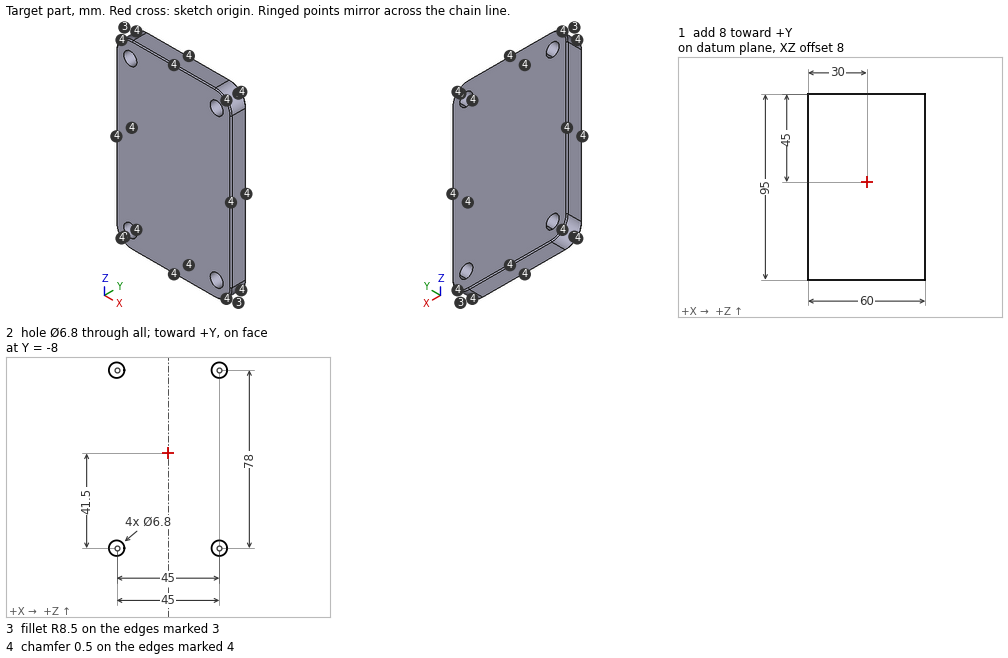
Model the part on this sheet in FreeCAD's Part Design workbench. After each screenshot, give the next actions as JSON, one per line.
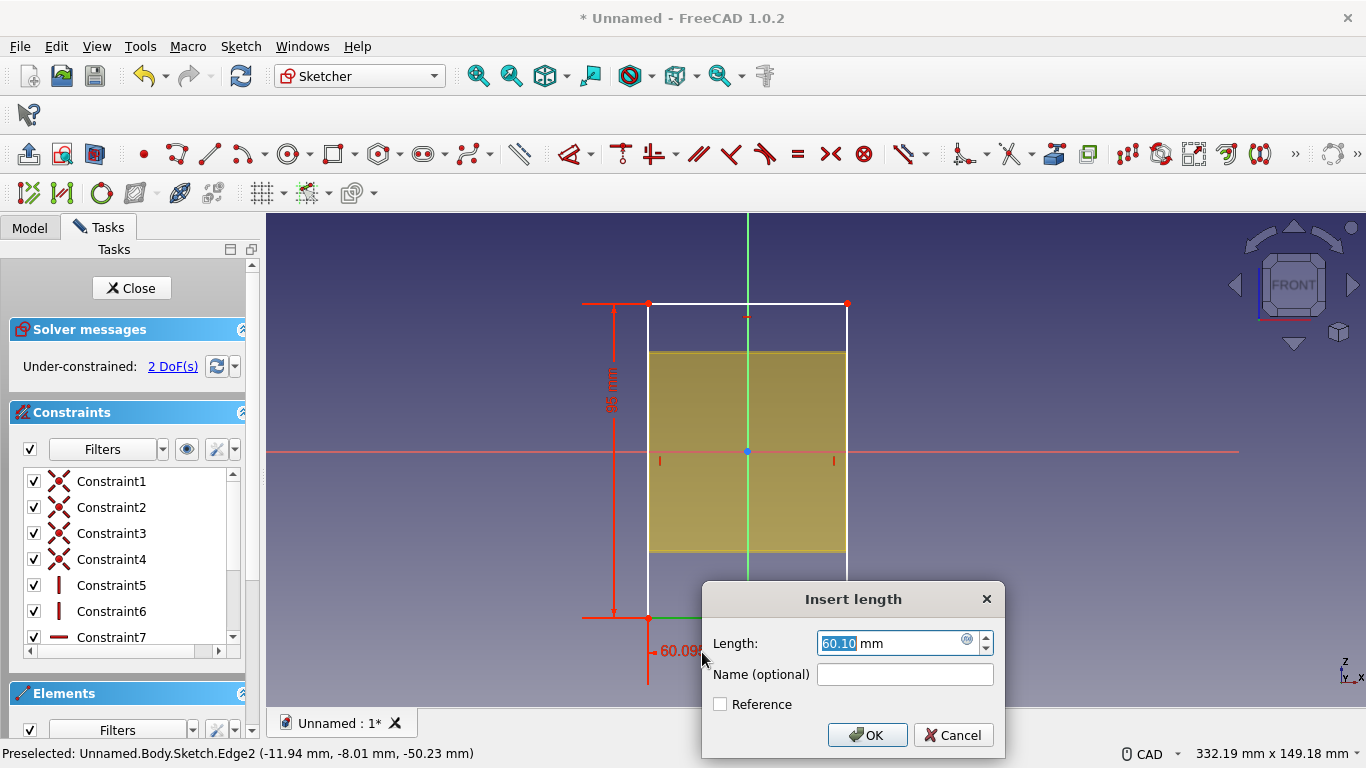
{"action": "type", "text": "60"}
{"action": "key", "text": "Return"}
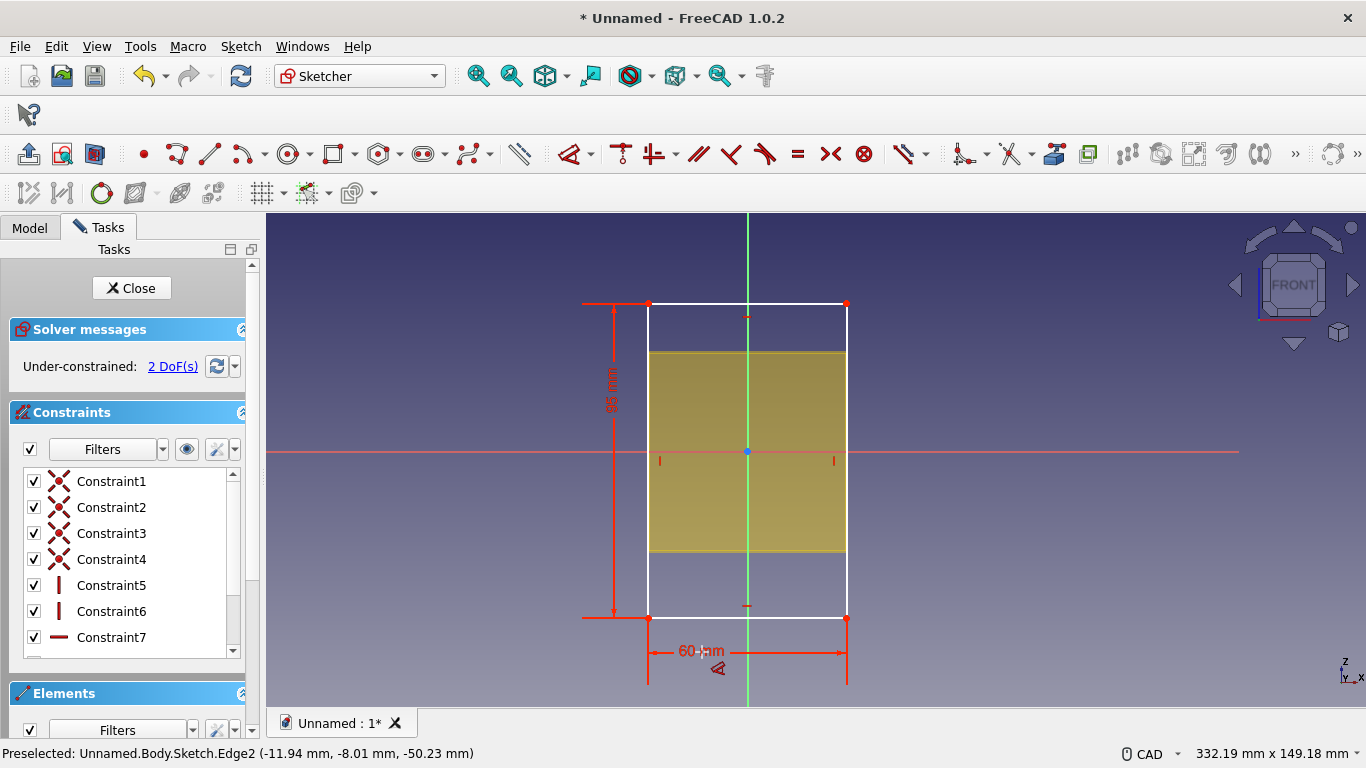
{"action": "left_click", "coordinate": [648, 304]}
{"action": "left_click", "coordinate": [698, 270]}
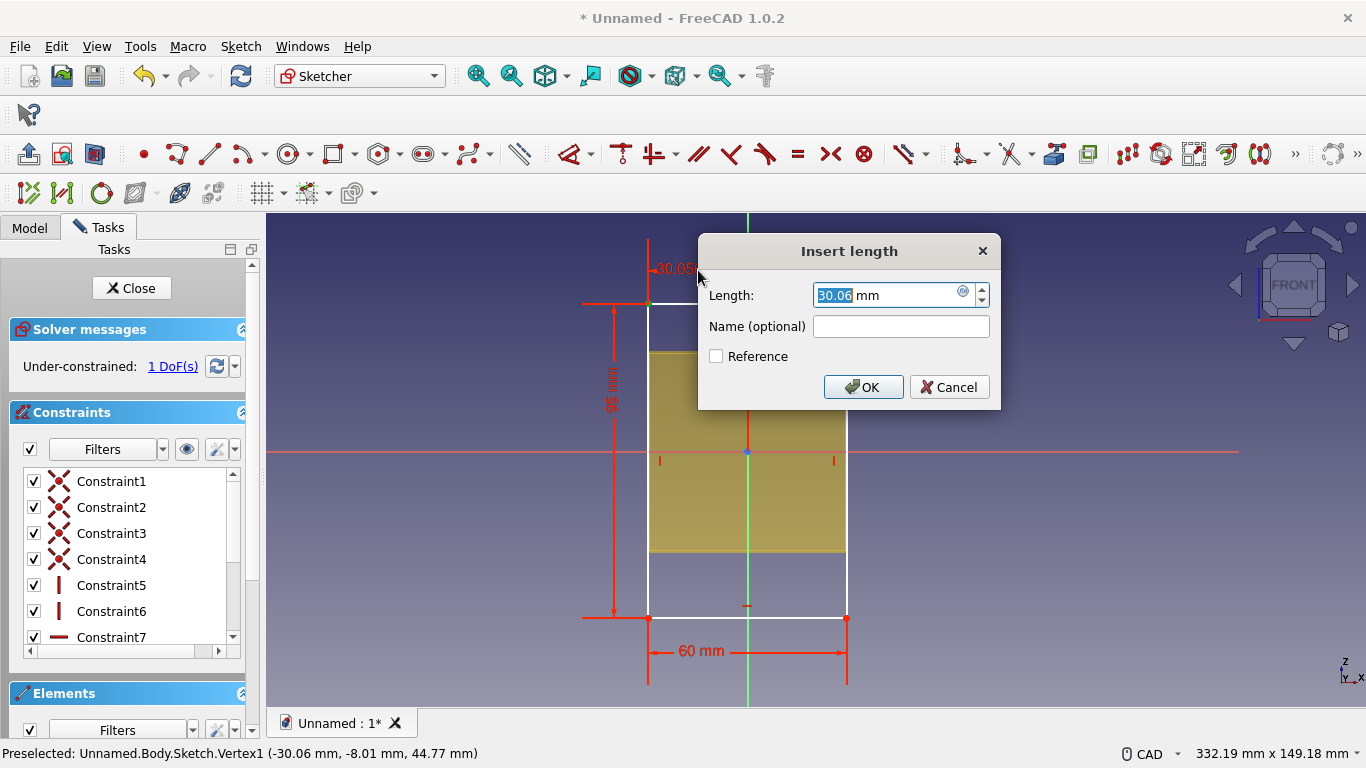
{"action": "type", "text": "30"}
{"action": "key", "text": "Return"}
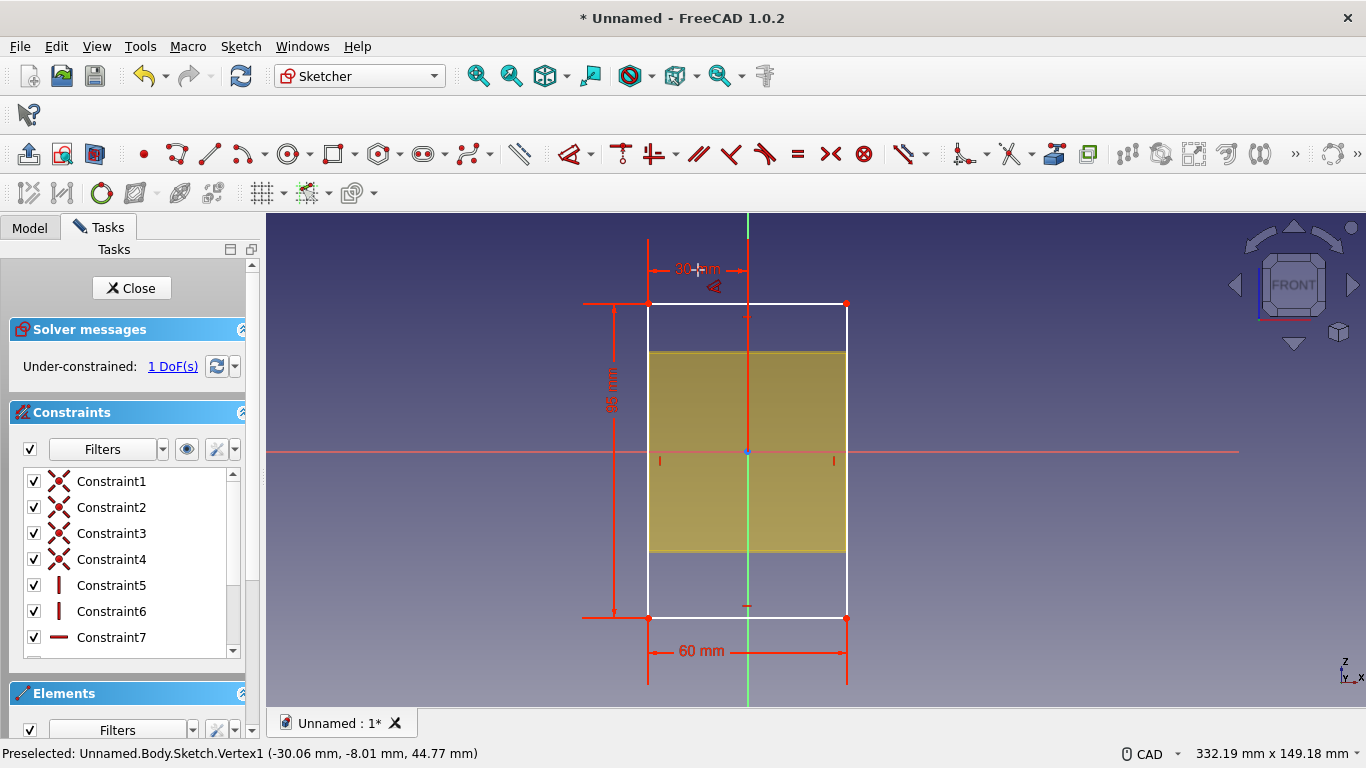
{"action": "left_click", "coordinate": [648, 304]}
{"action": "left_click", "coordinate": [614, 344]}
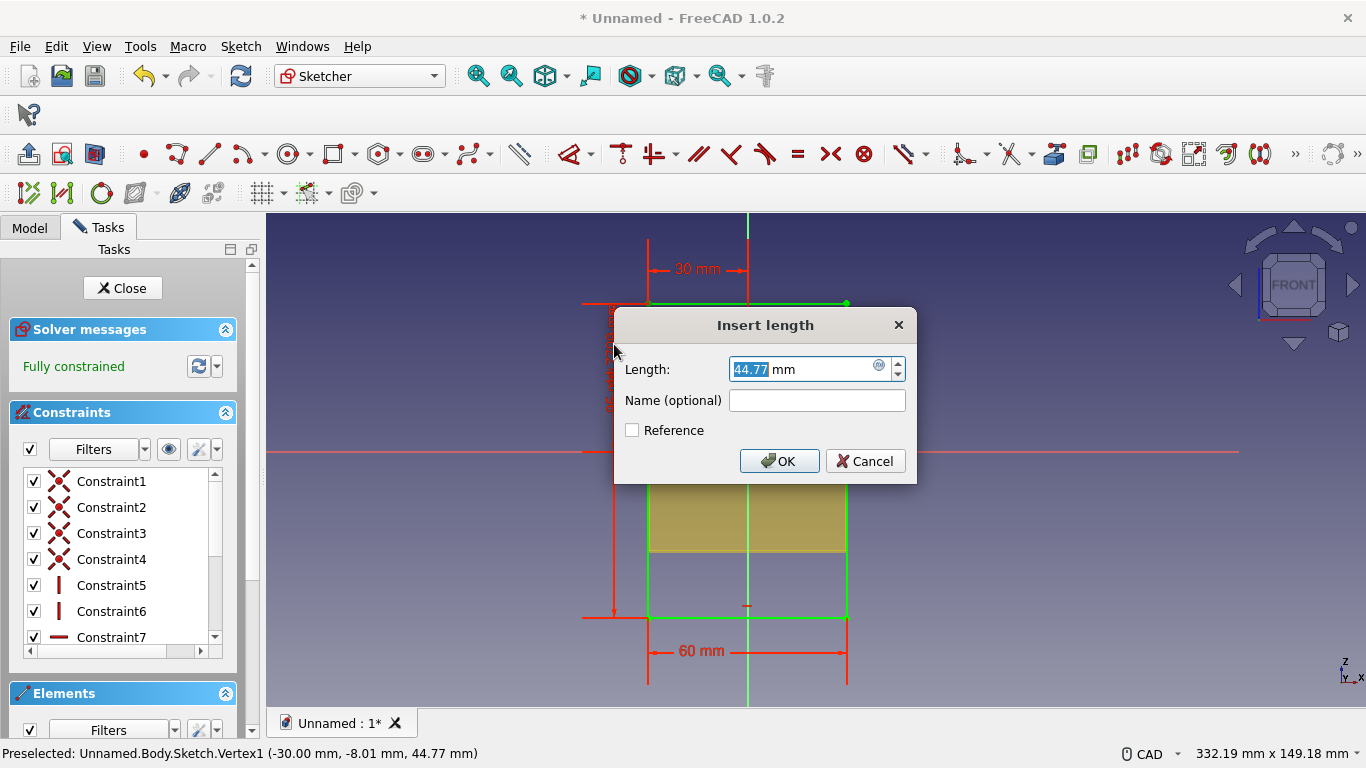
{"action": "type", "text": "45"}
{"action": "key", "text": "Return"}
{"action": "key", "text": "Escape"}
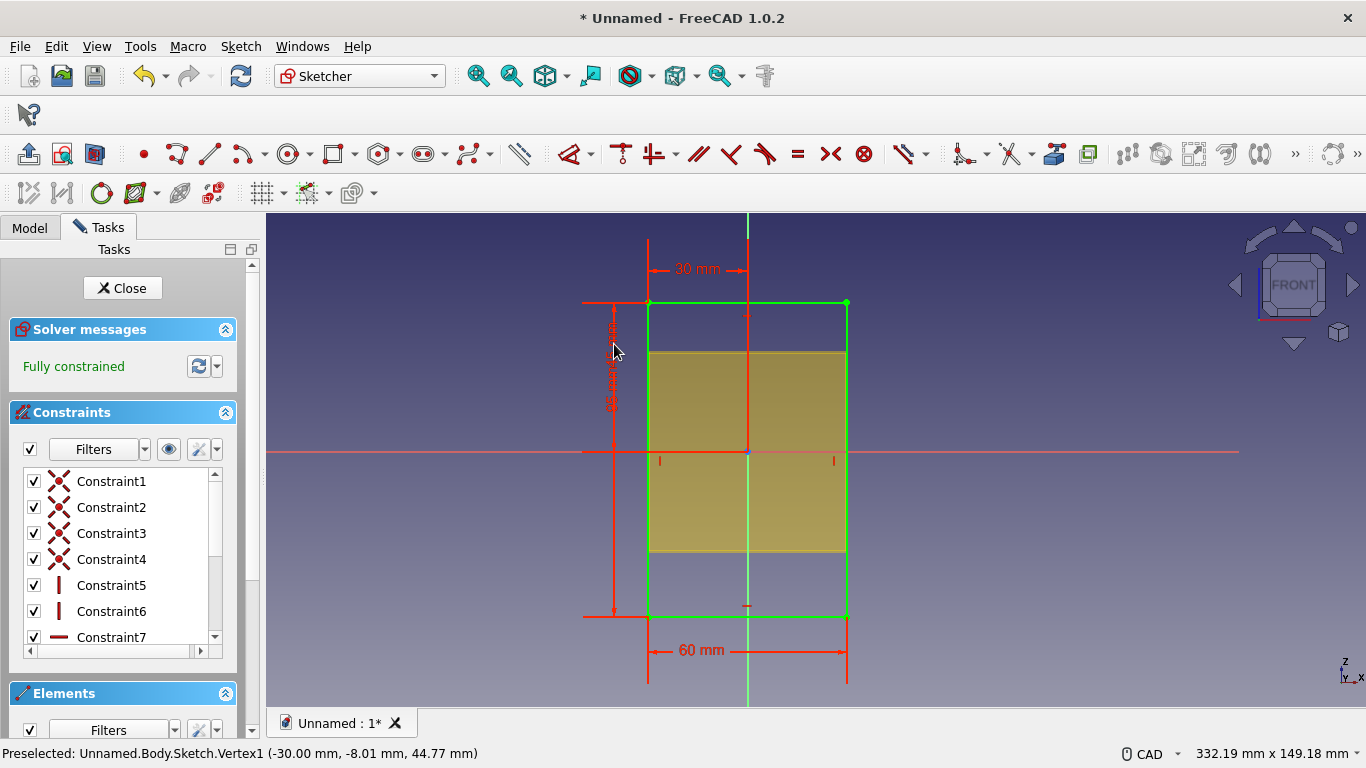
{"action": "left_click", "coordinate": [123, 288]}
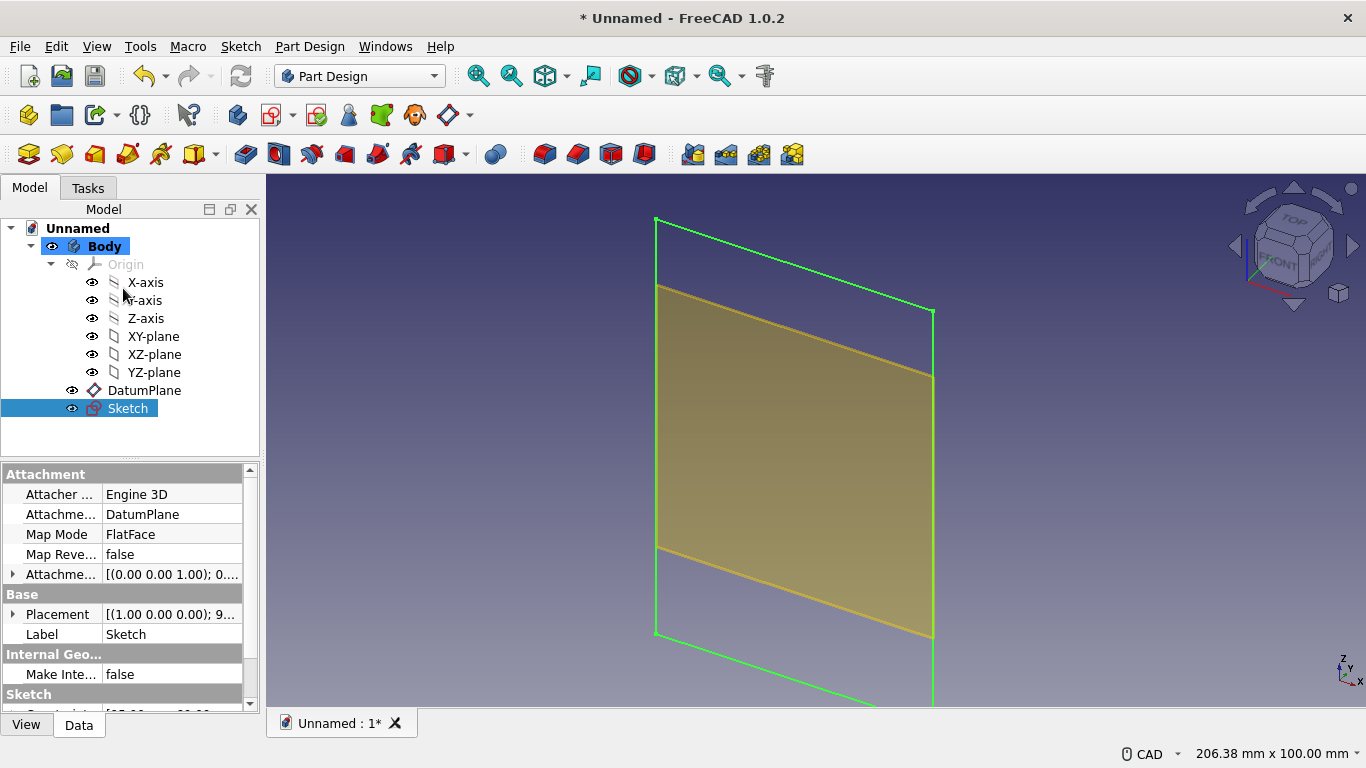
{"action": "left_click", "coordinate": [29, 154]}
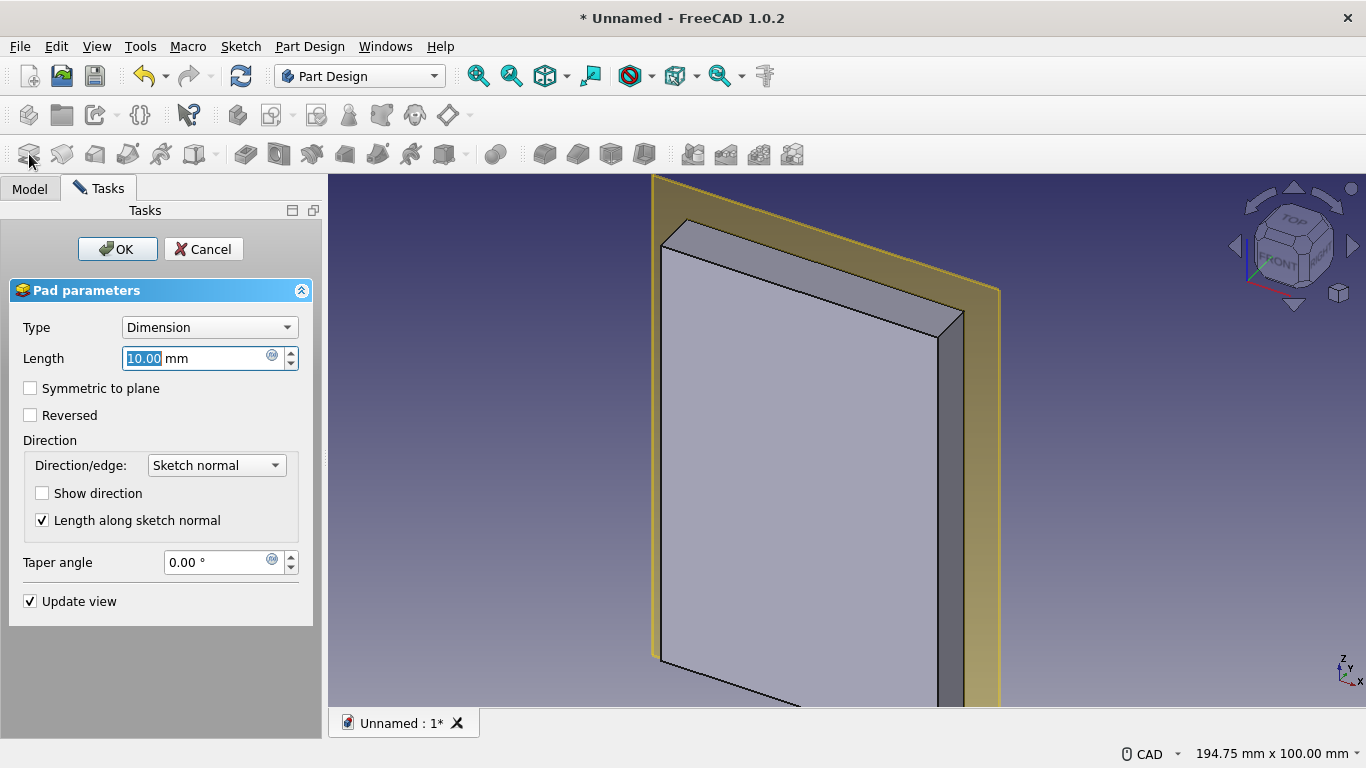
{"action": "type", "text": "8"}
{"action": "key", "text": "Tab"}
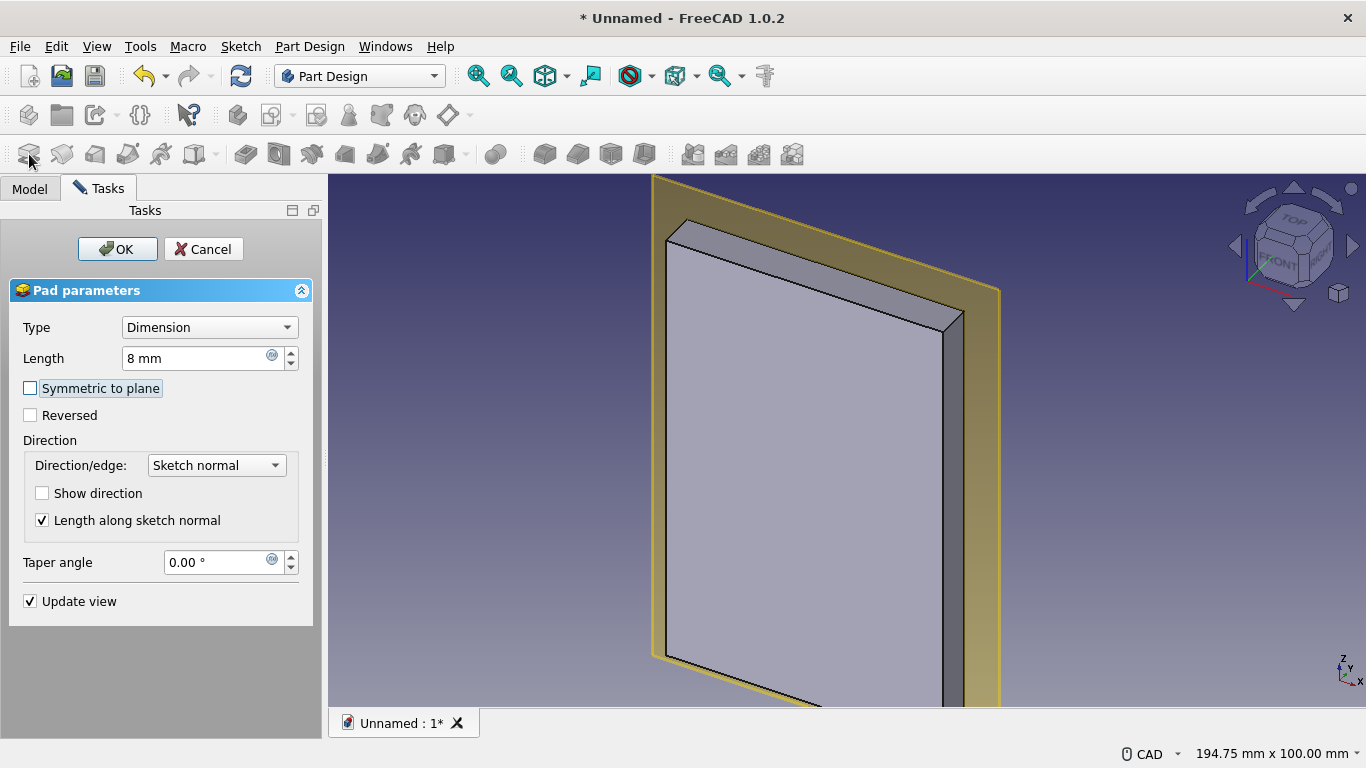
{"action": "left_click", "coordinate": [31, 415]}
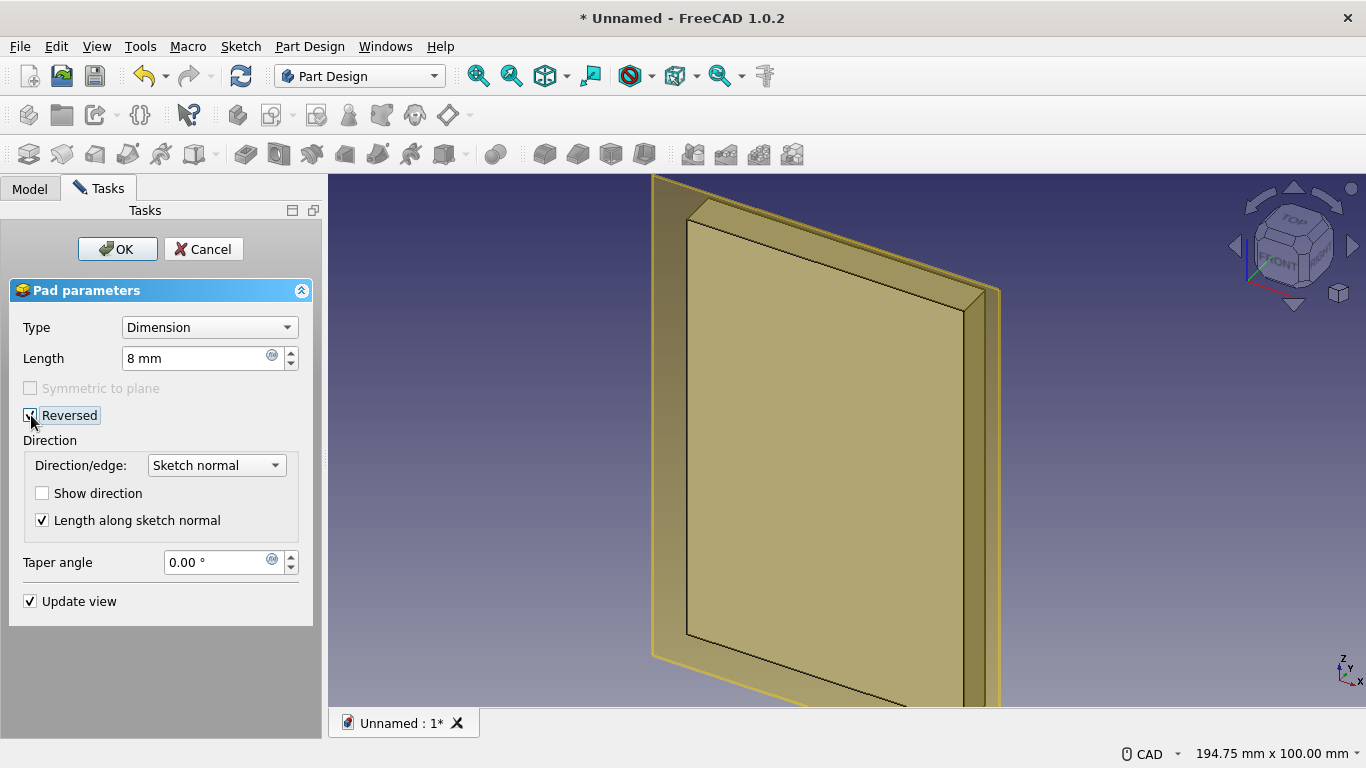
{"action": "left_click", "coordinate": [118, 249]}